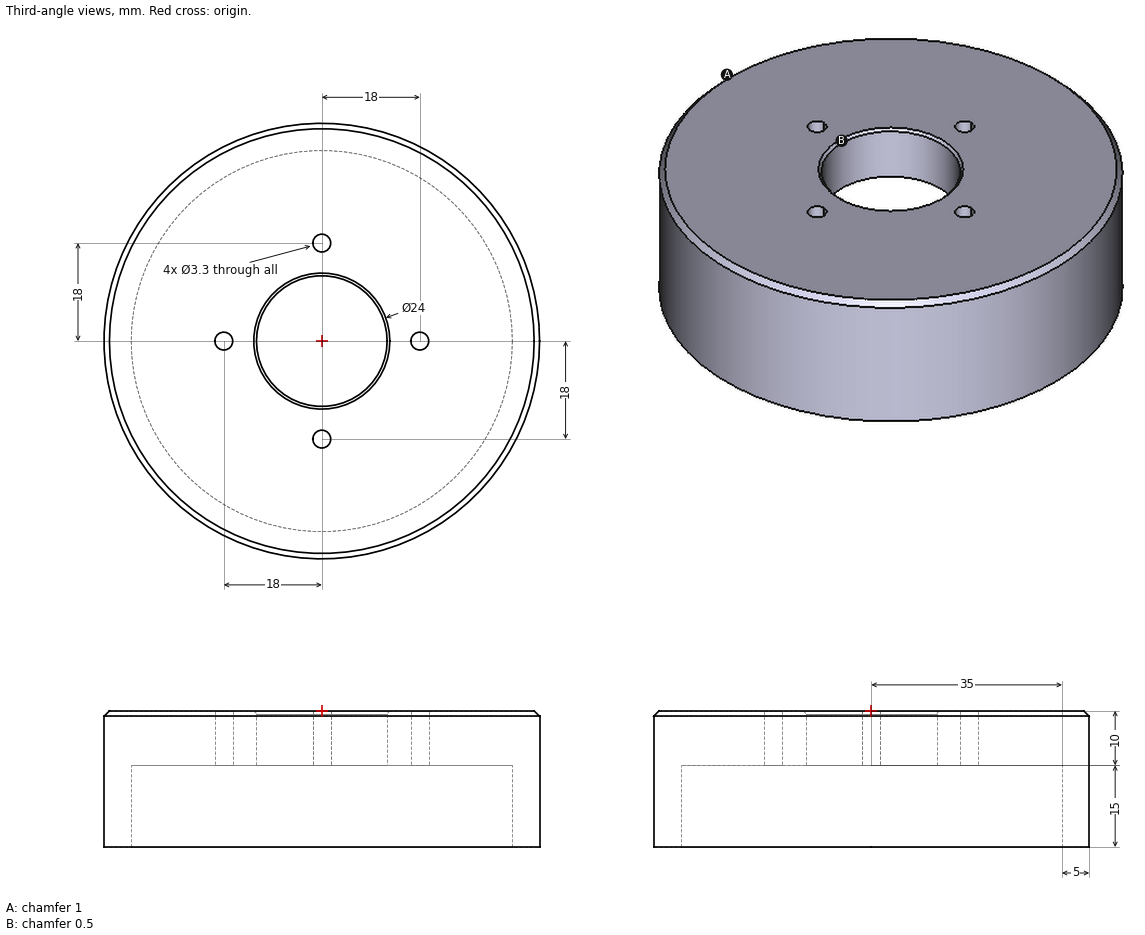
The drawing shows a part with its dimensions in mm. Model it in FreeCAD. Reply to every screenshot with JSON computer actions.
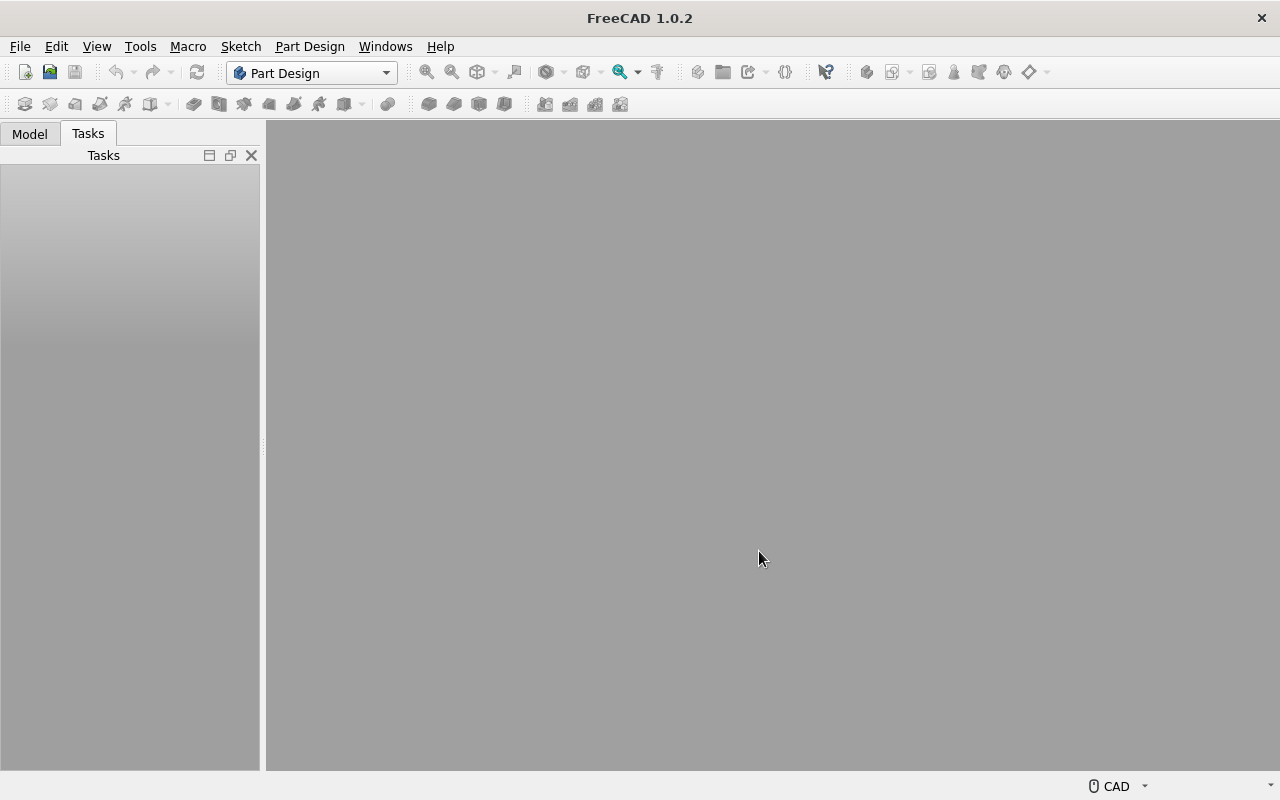
{"action": "key", "text": "ctrl+n"}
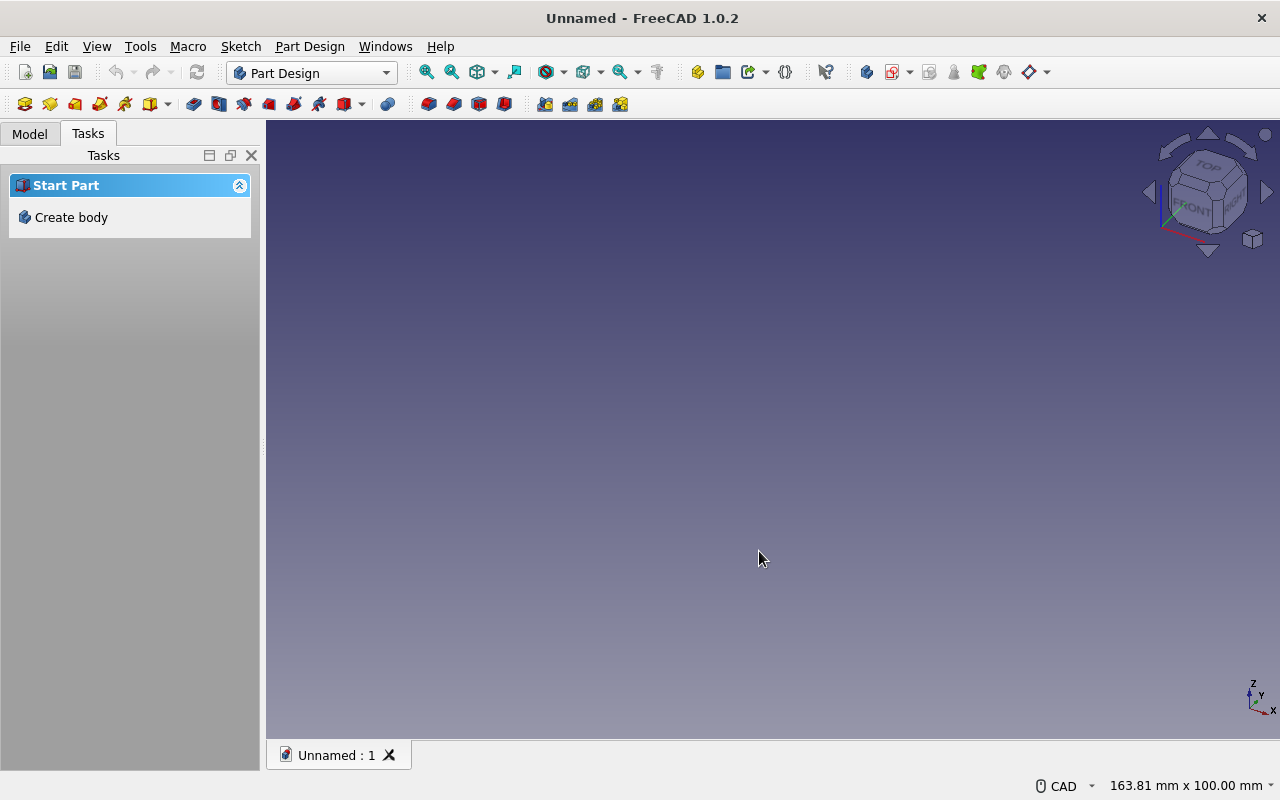
{"action": "left_click", "coordinate": [892, 72]}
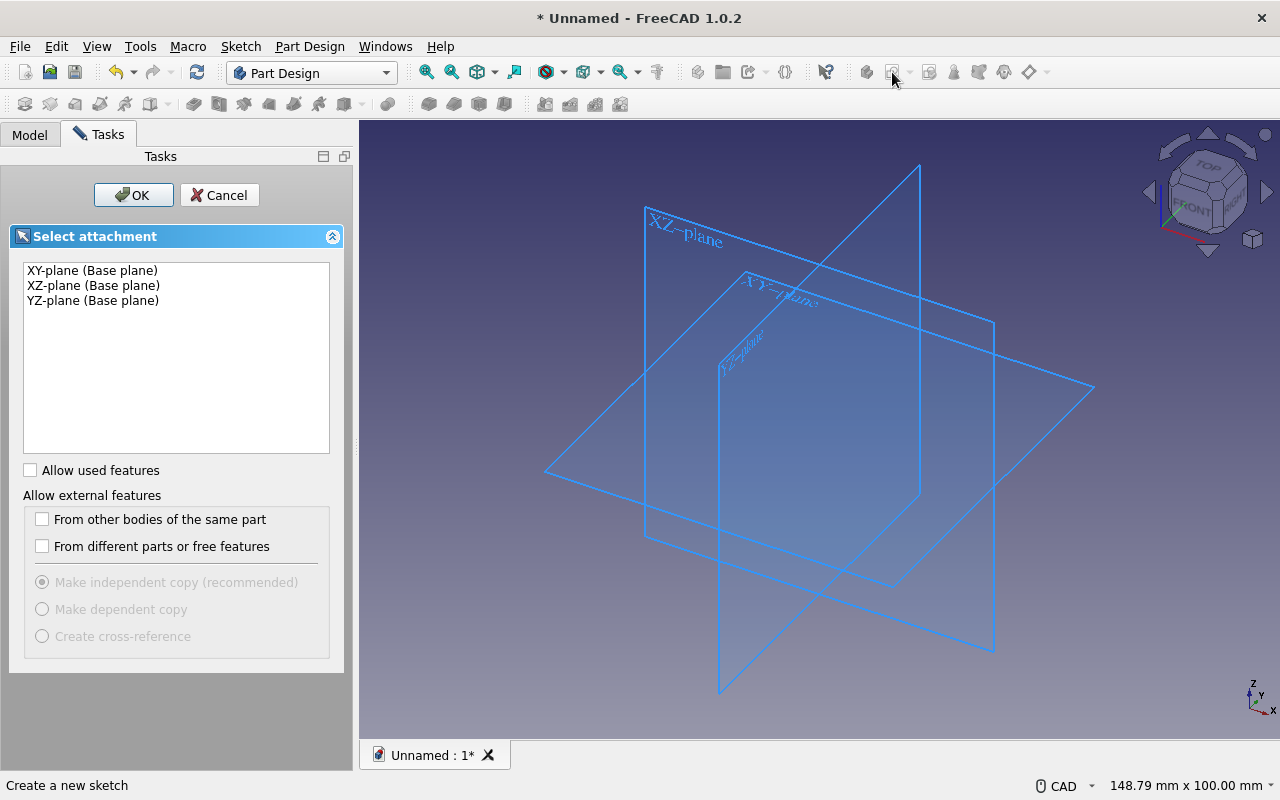
{"action": "left_click", "coordinate": [84, 300]}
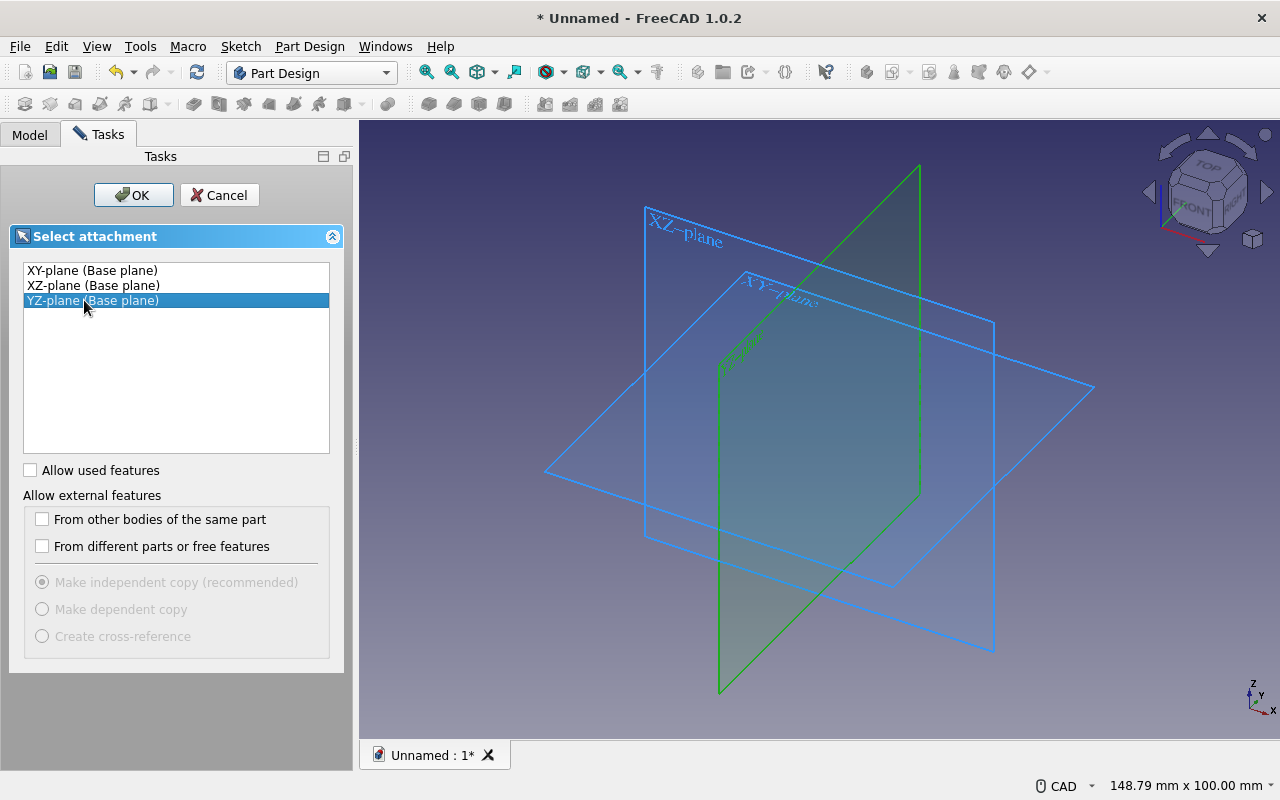
{"action": "left_click", "coordinate": [134, 195]}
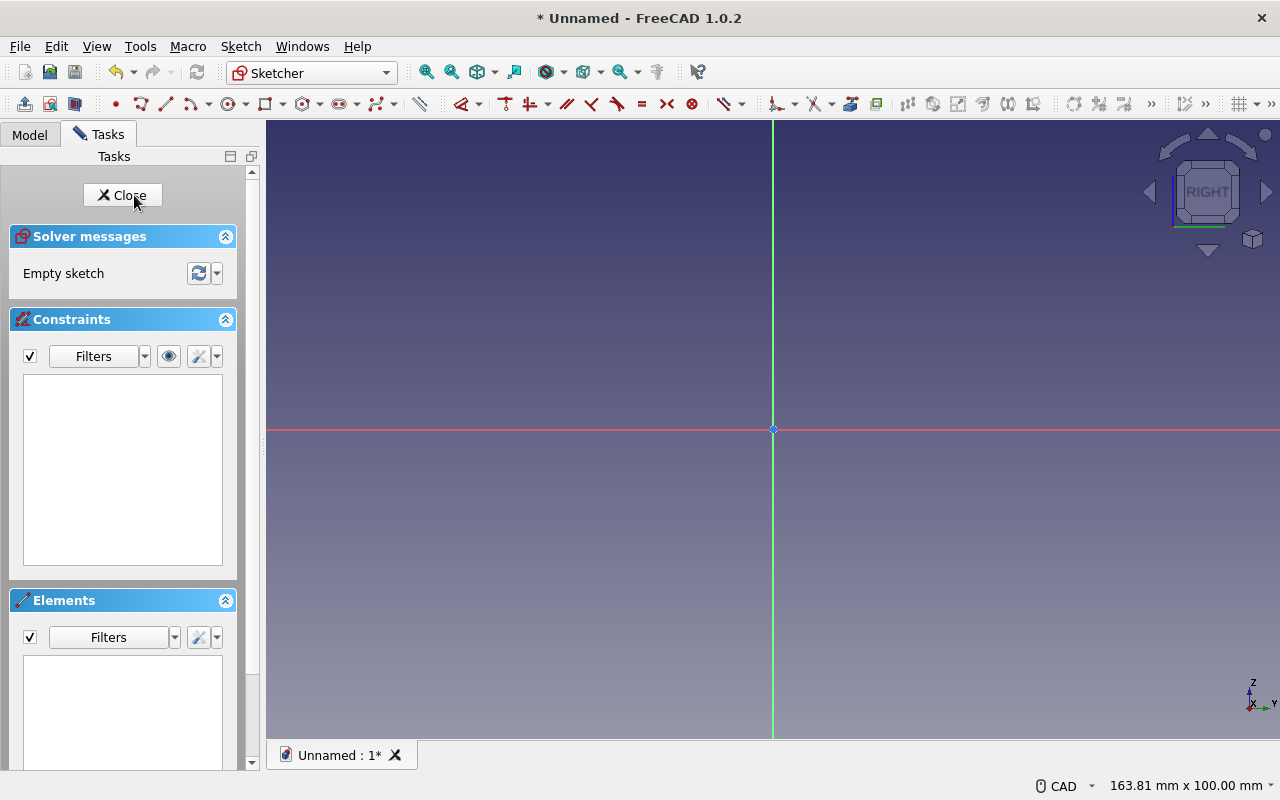
{"action": "scroll", "coordinate": [1054, 570], "scroll_direction": "up", "scroll_amount": 4}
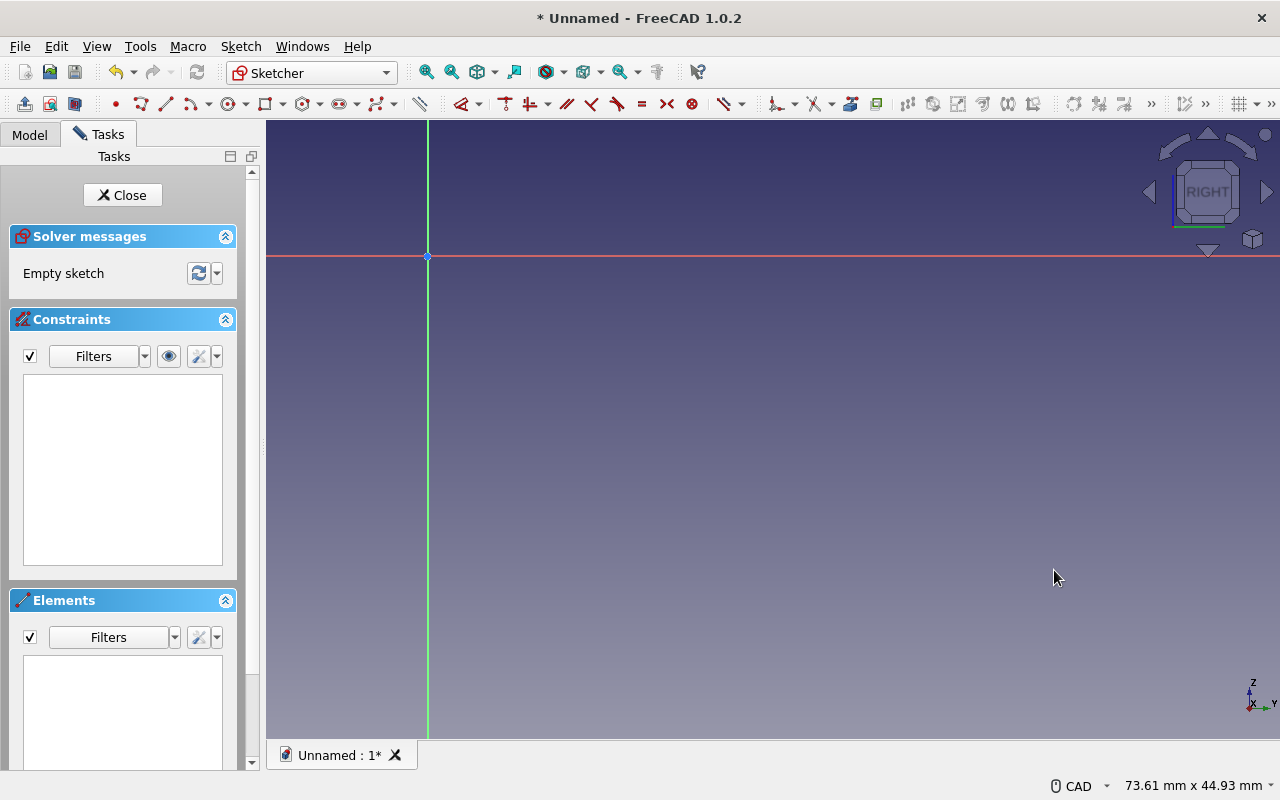
{"action": "key", "text": "g m"}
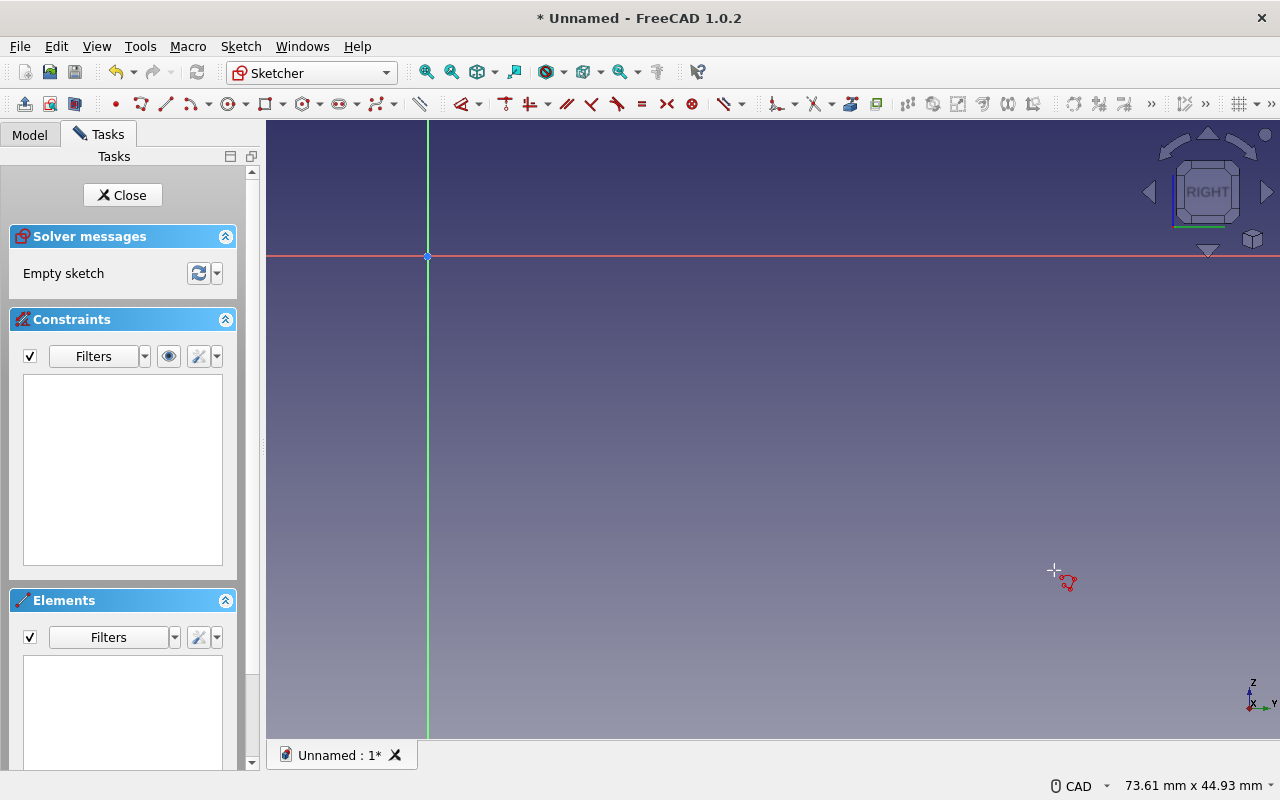
{"action": "left_click", "coordinate": [428, 256]}
{"action": "left_click", "coordinate": [437, 394]}
{"action": "left_click", "coordinate": [910, 394]}
{"action": "left_click", "coordinate": [910, 601]}
{"action": "left_click", "coordinate": [979, 601]}
{"action": "left_click", "coordinate": [979, 265]}
{"action": "left_click", "coordinate": [428, 256]}
{"action": "key", "text": "Escape"}
{"action": "key", "text": "Escape"}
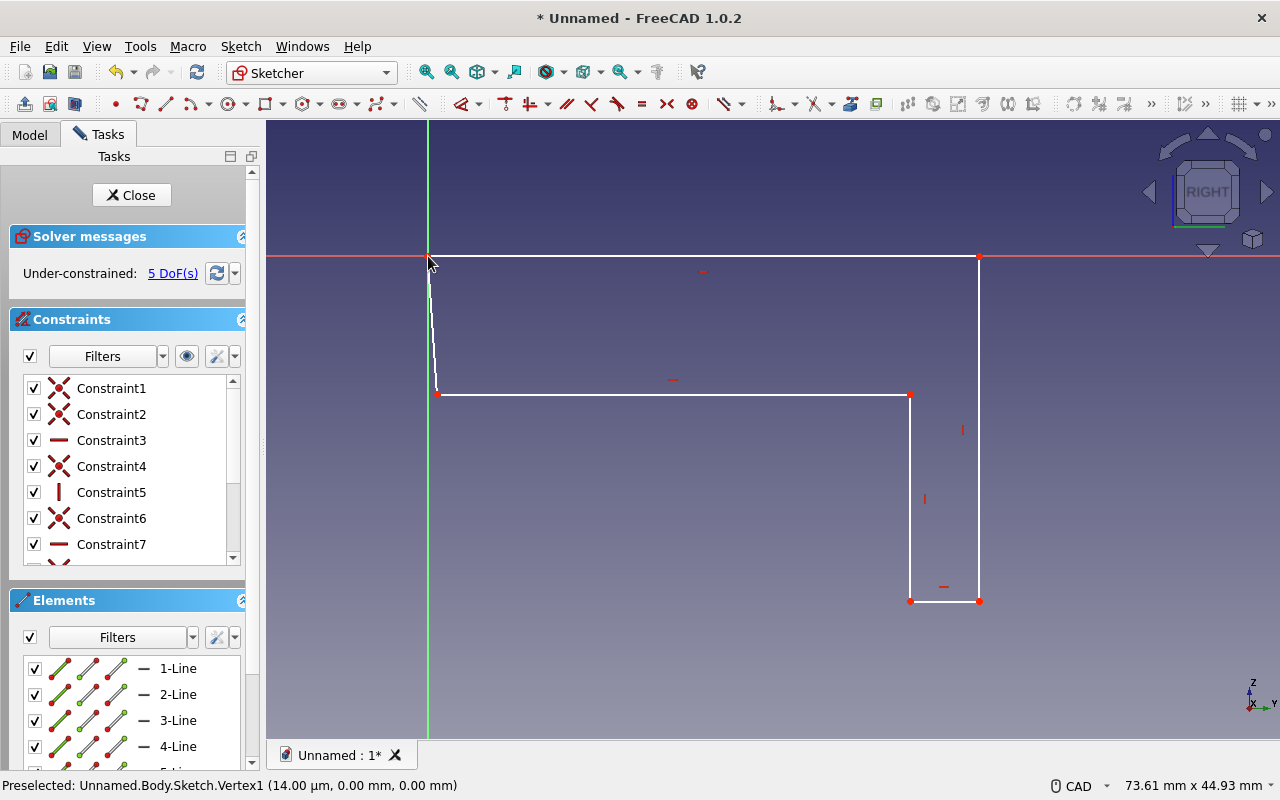
{"action": "left_click", "coordinate": [430, 298]}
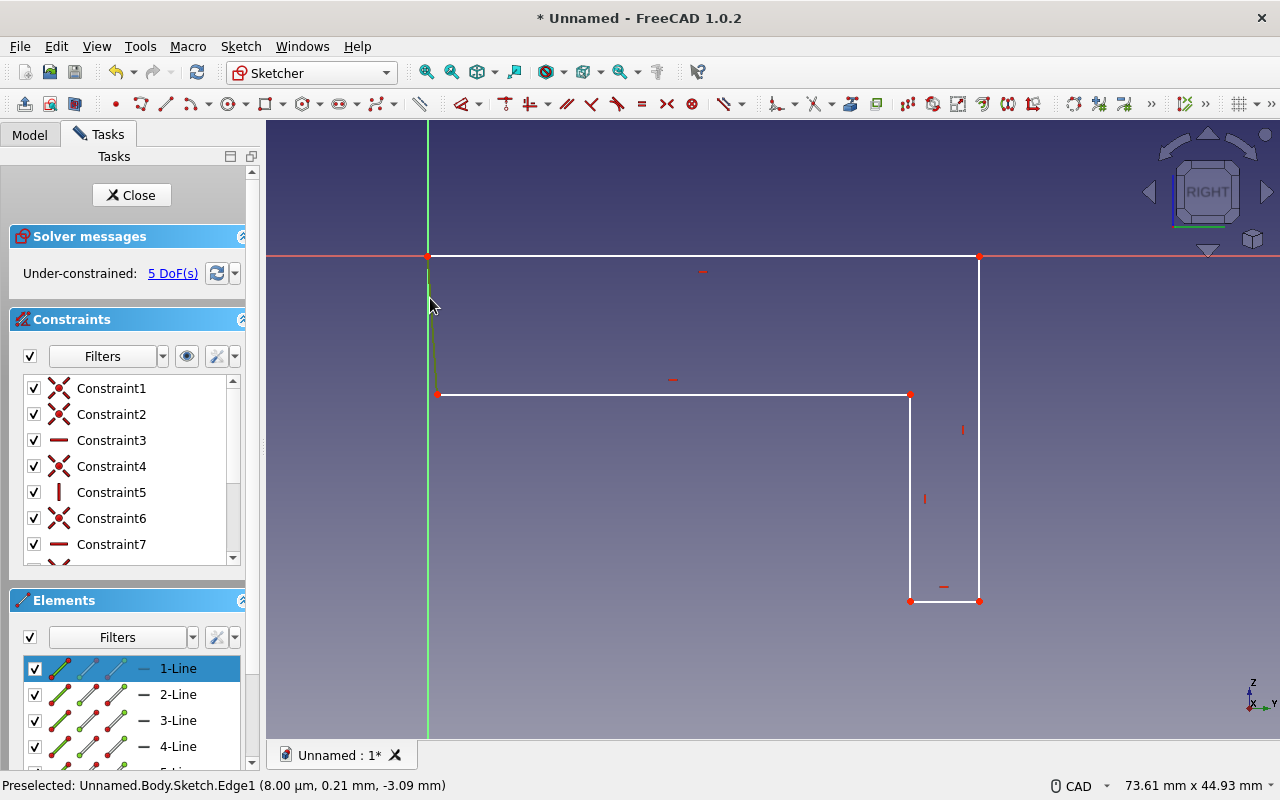
{"action": "key", "text": "v"}